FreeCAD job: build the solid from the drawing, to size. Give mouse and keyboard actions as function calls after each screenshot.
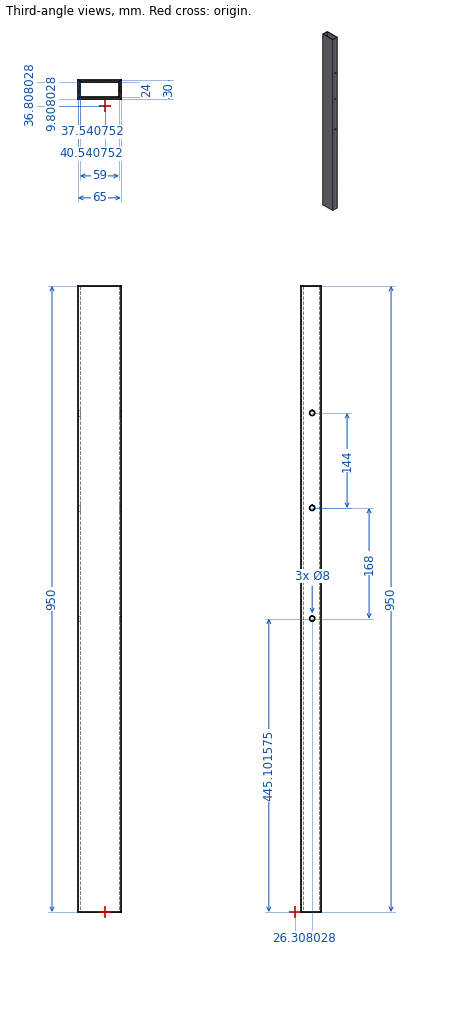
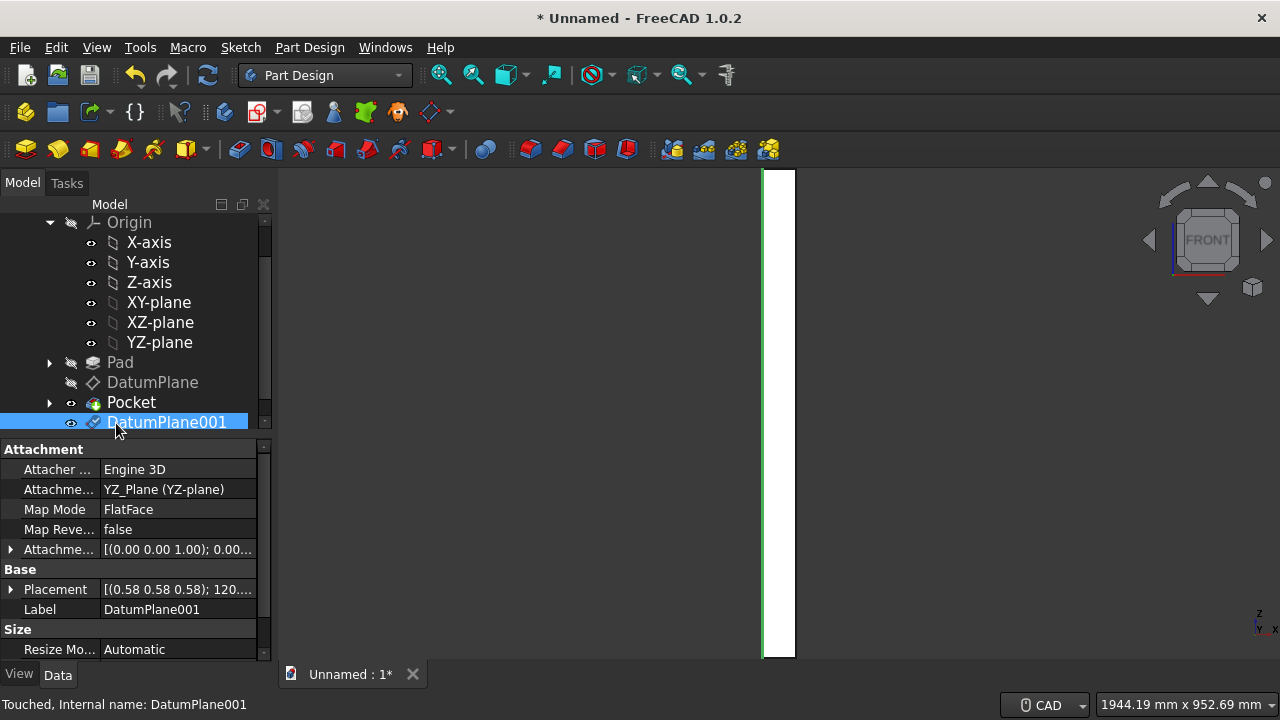
click(258, 112)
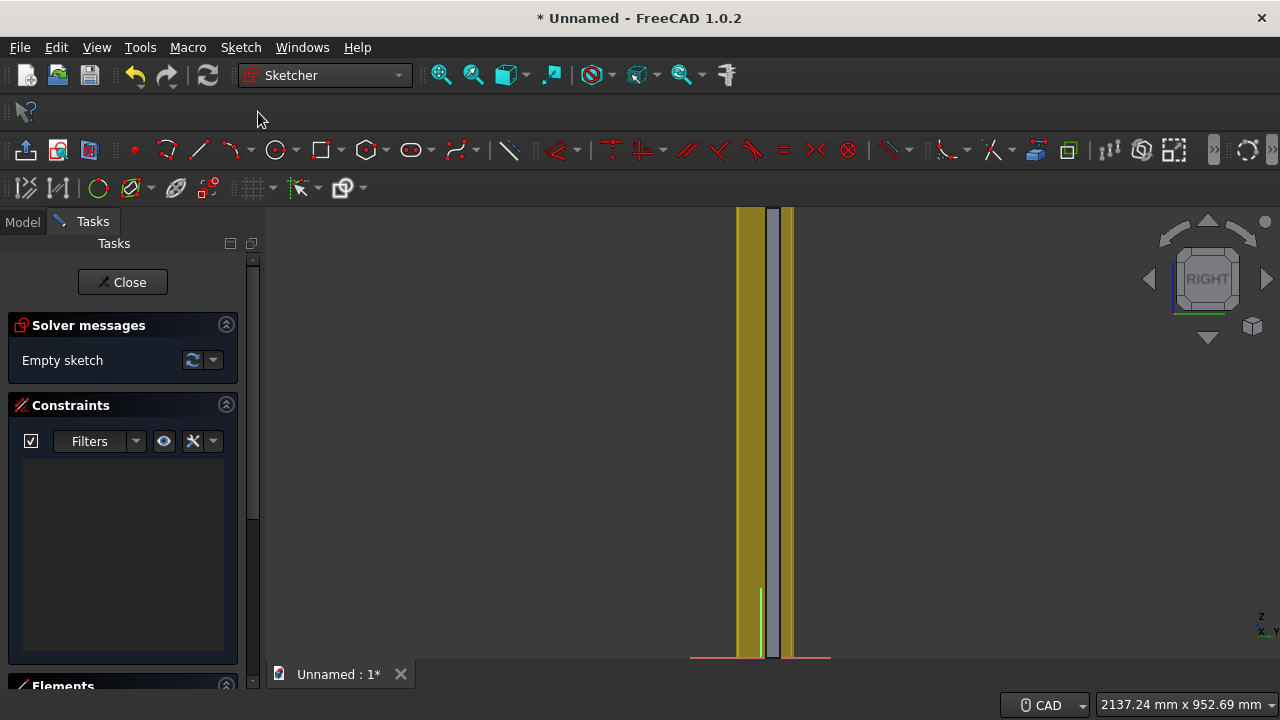
click(90, 150)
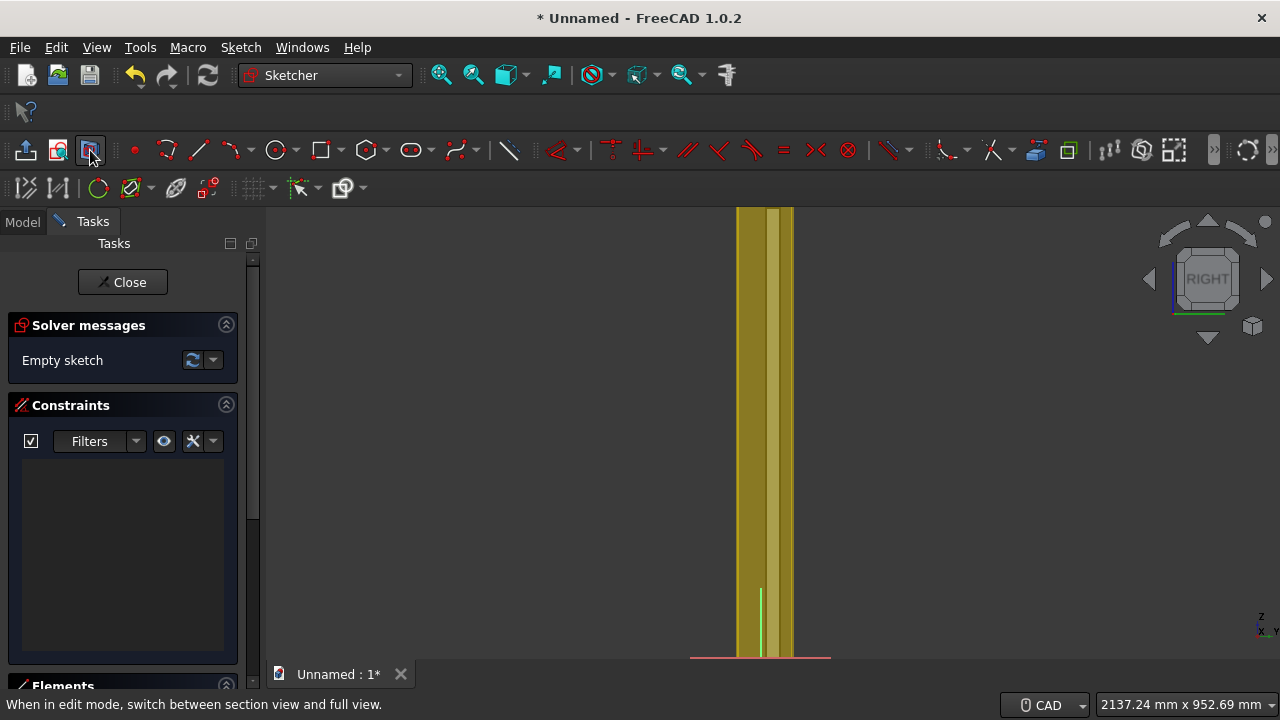
scroll(416, 235, down, 1)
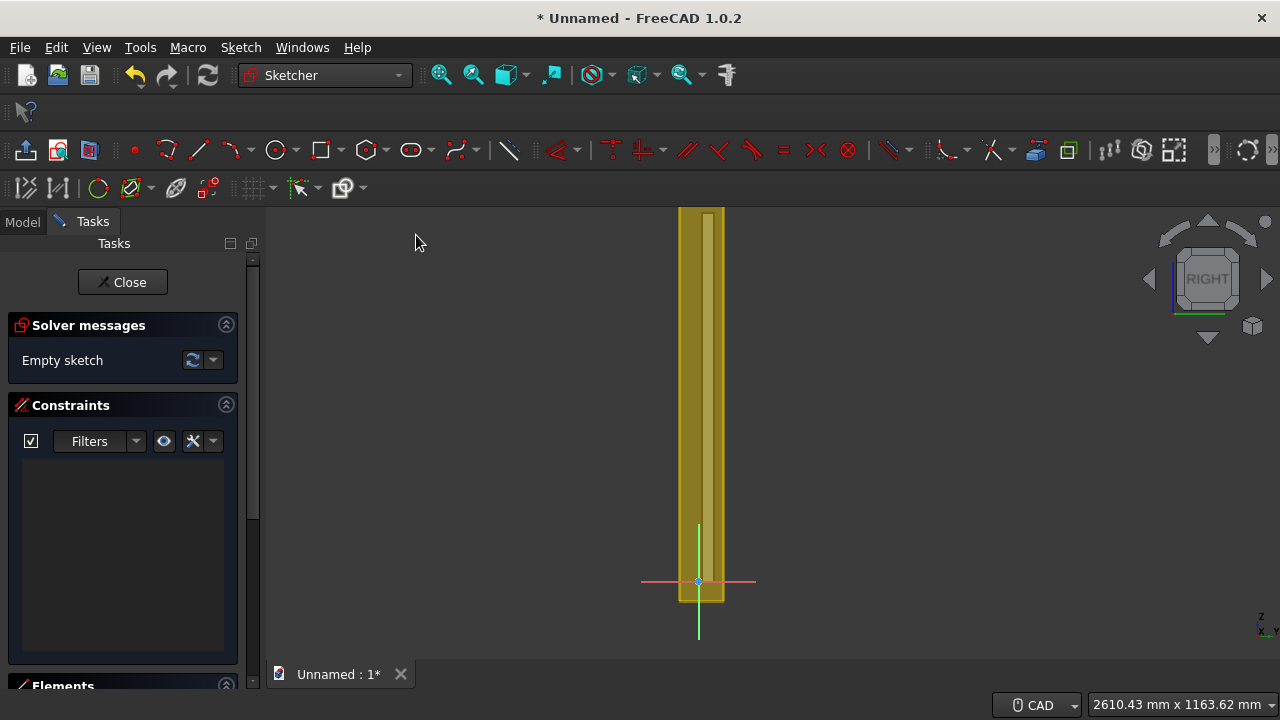
click(276, 150)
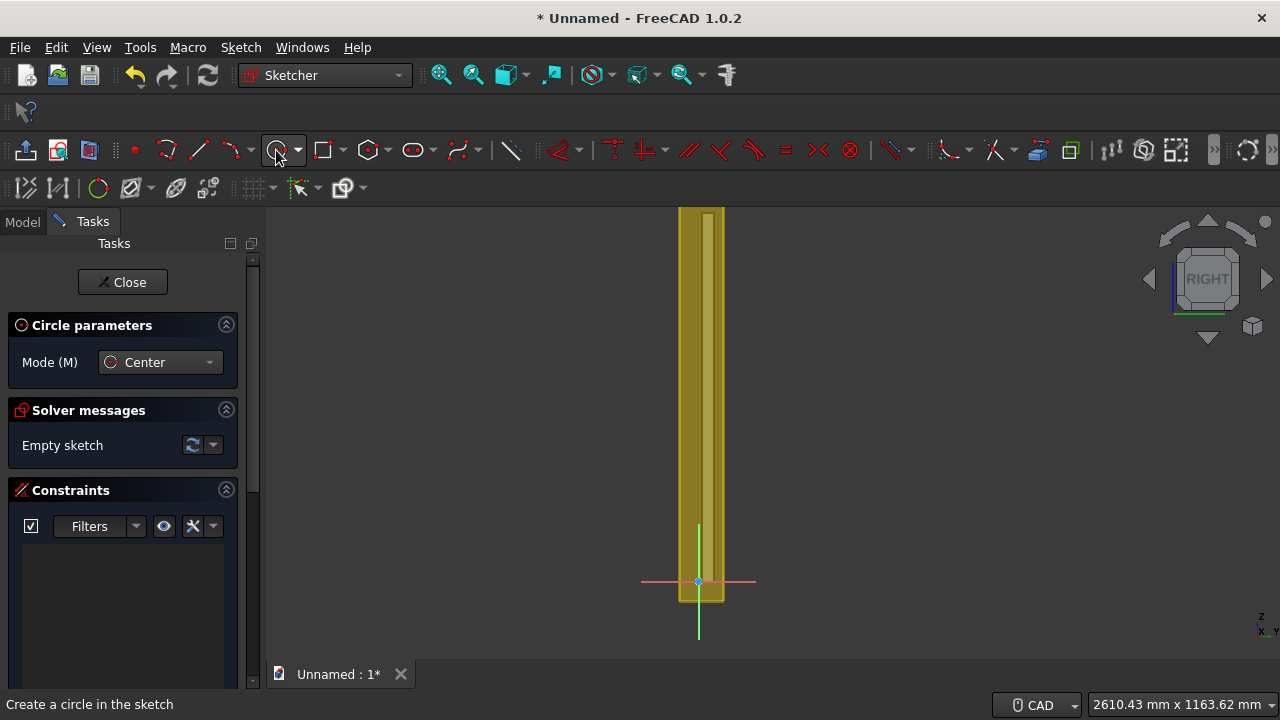
scroll(709, 409, up, 14)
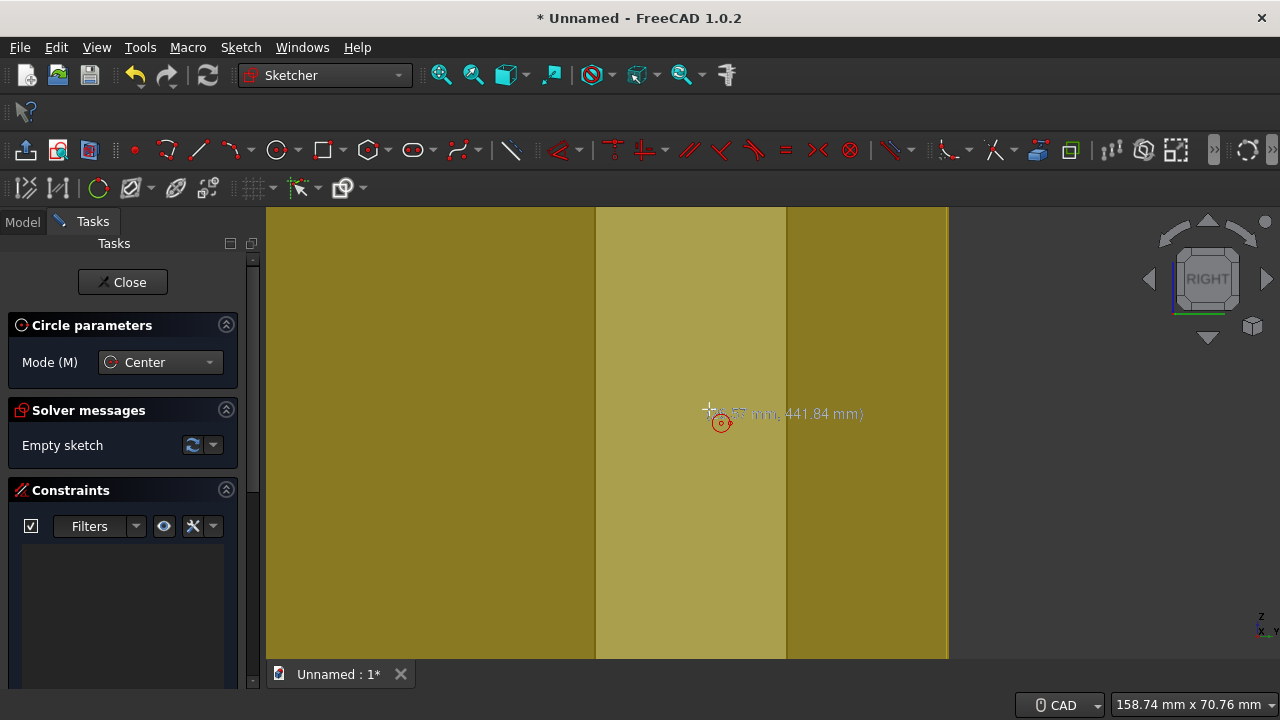
scroll(709, 409, down, 14)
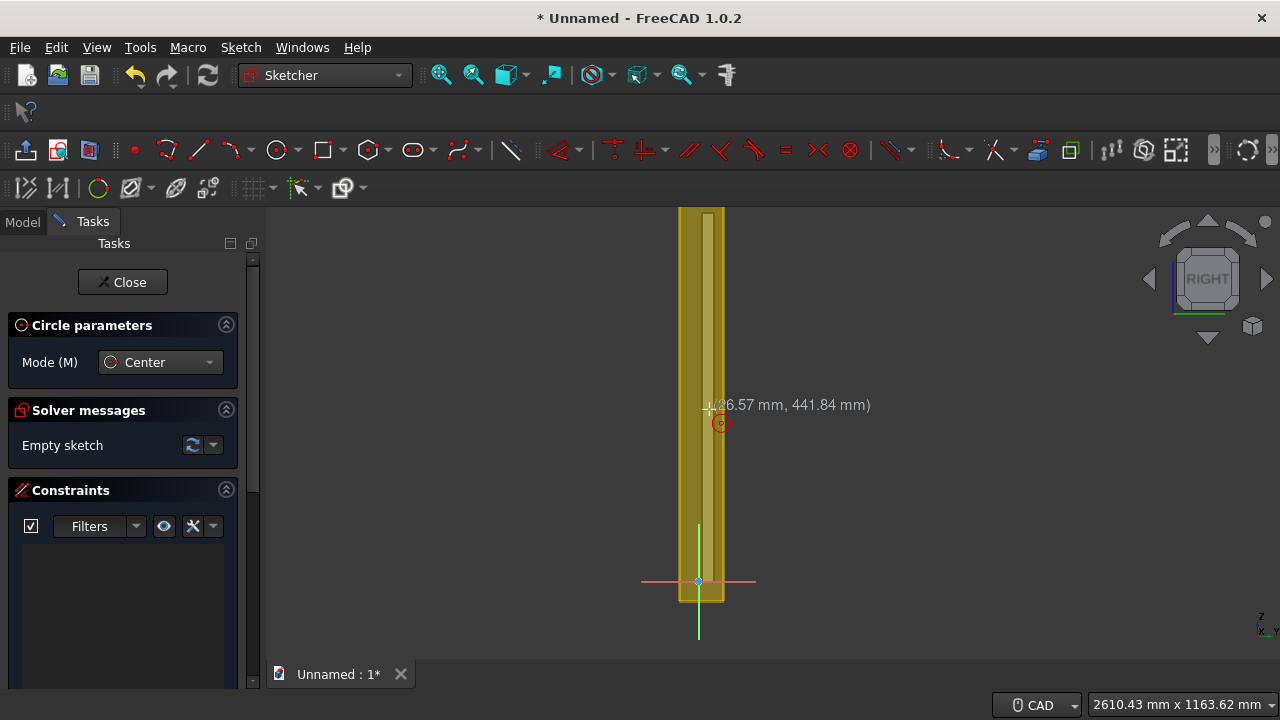
scroll(709, 409, up, 3)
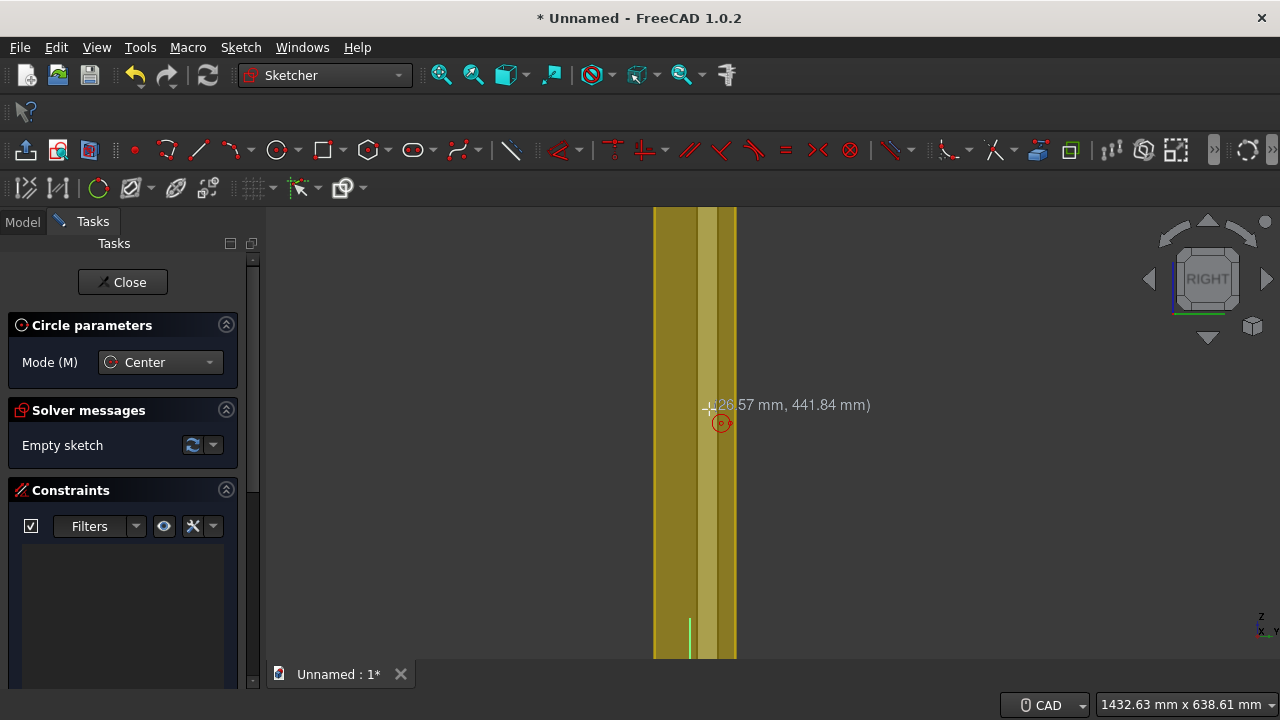
click(708, 408)
move(710, 406)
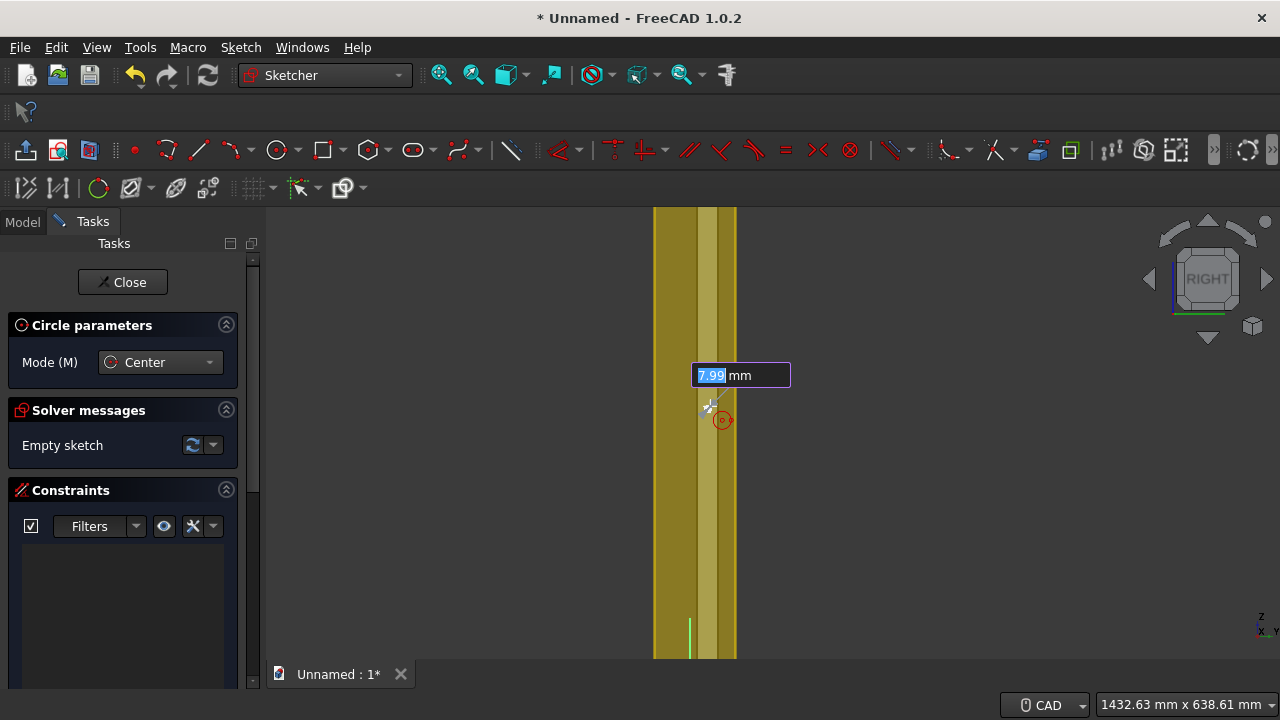
text(8)
key(Return)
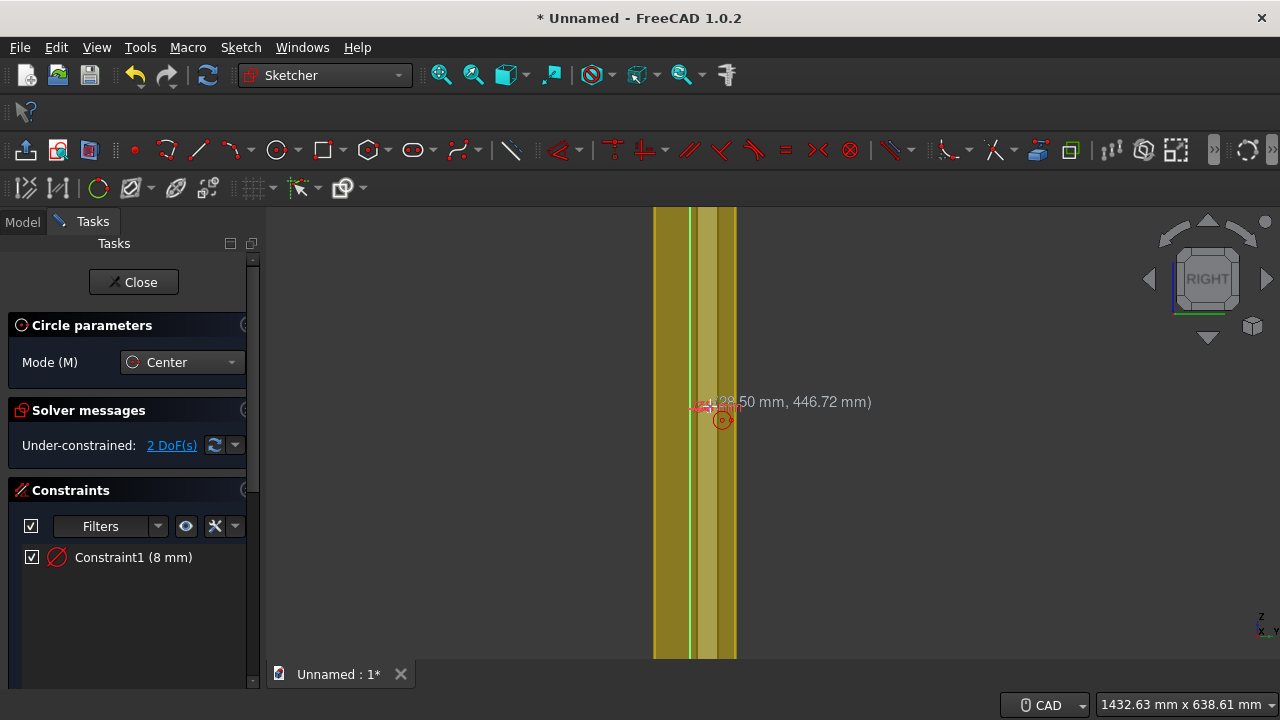
scroll(708, 289, up, 11)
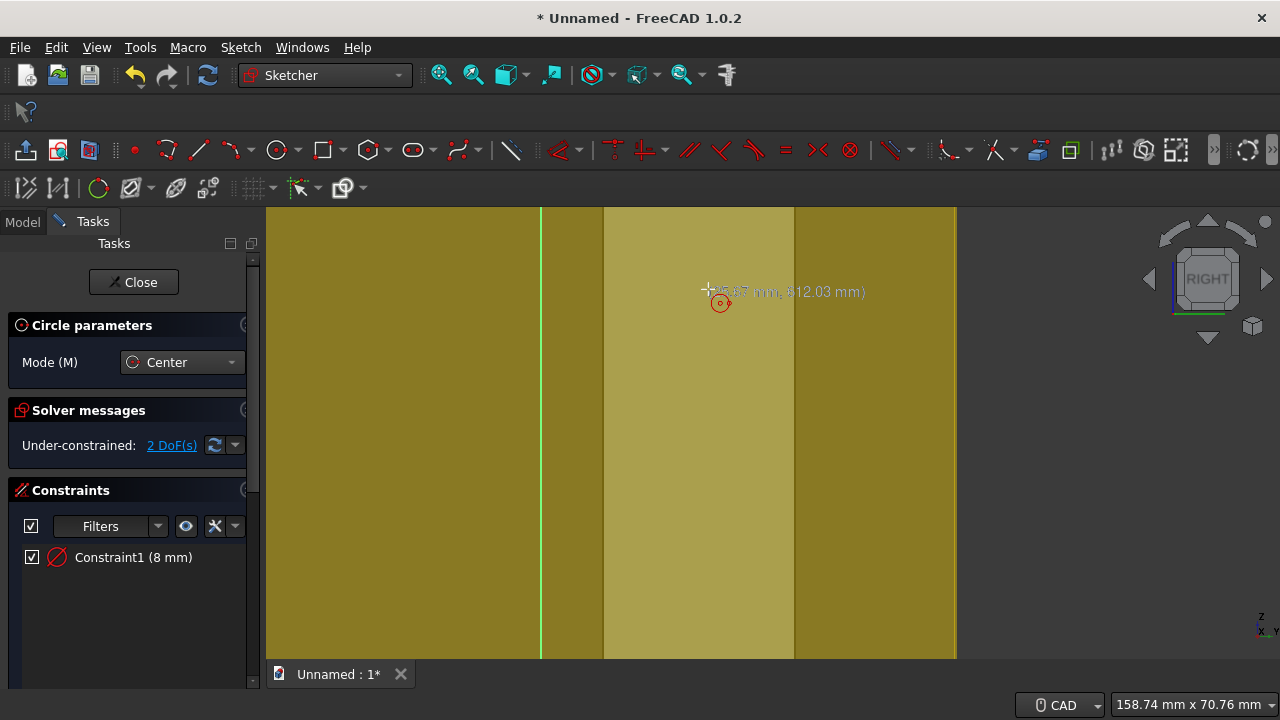
scroll(709, 346, down, 14)